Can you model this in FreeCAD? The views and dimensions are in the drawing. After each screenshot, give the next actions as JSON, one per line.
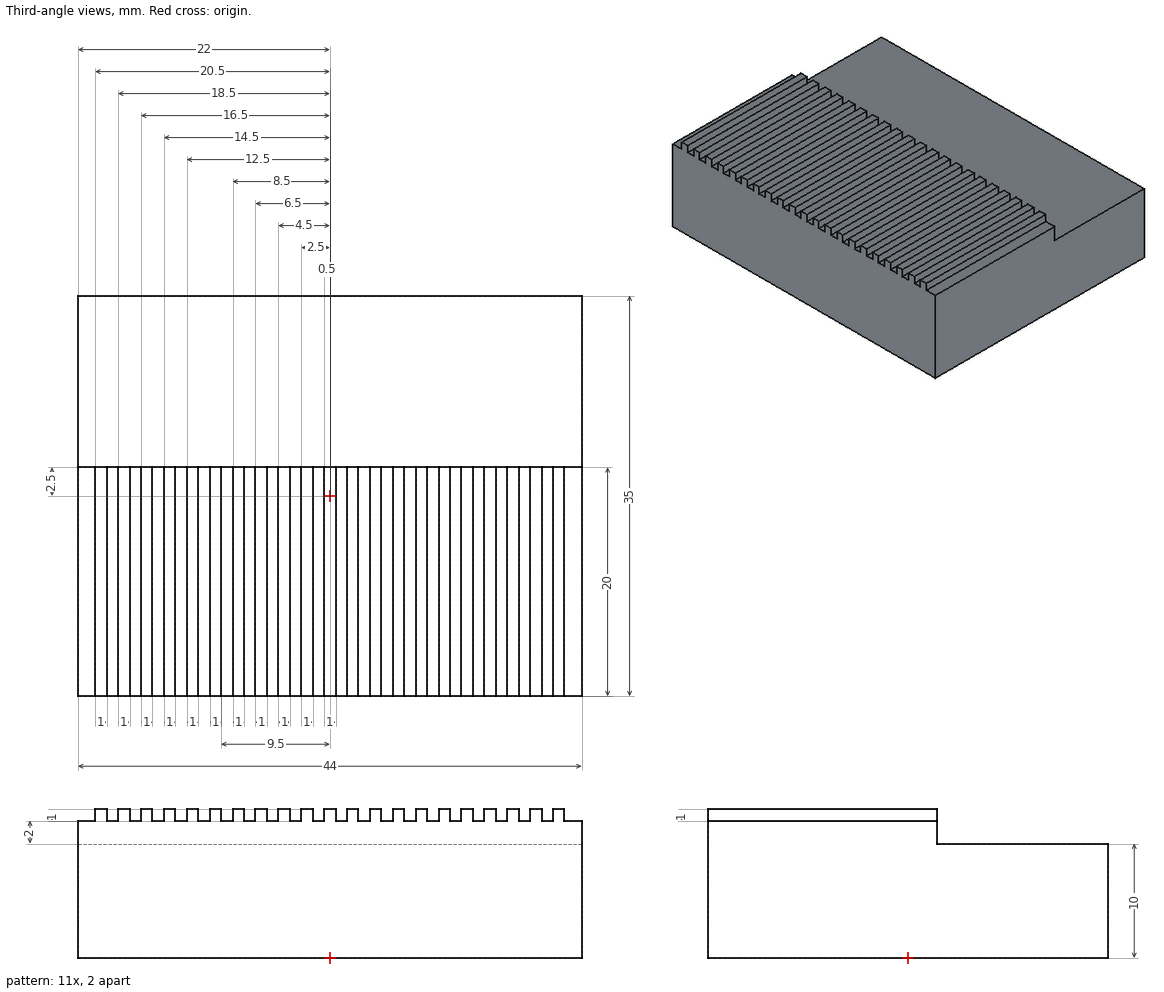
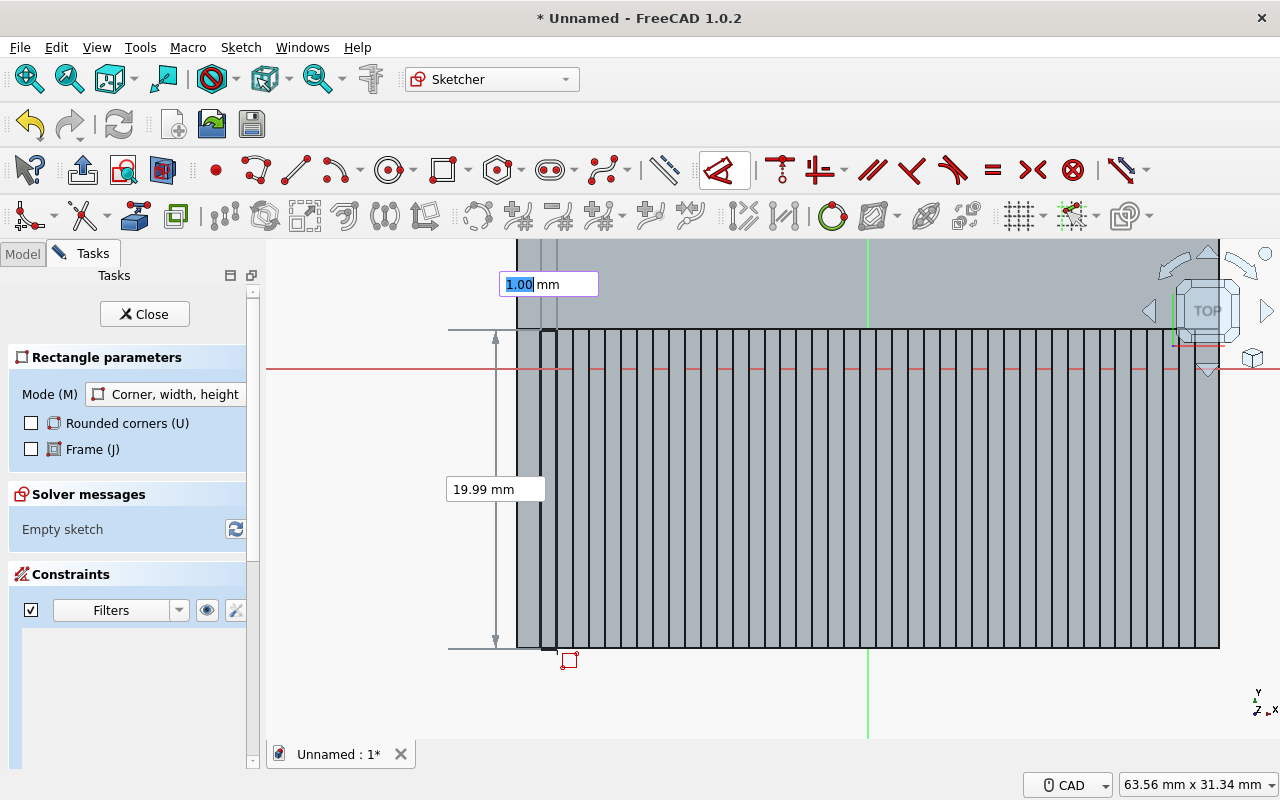
{"action": "type", "text": "1"}
{"action": "key", "text": "Tab"}
{"action": "type", "text": "20"}
{"action": "key", "text": "Return"}
{"action": "key", "text": "Escape"}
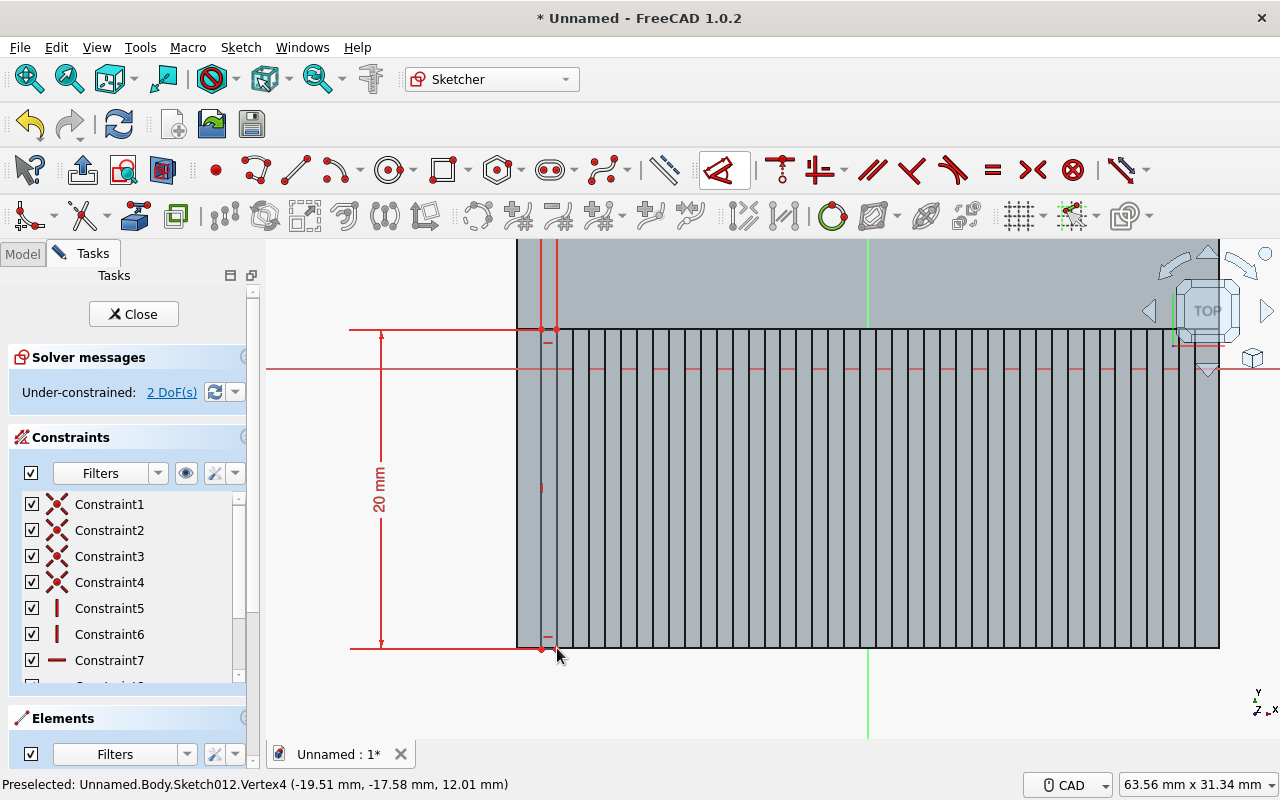
{"action": "left_click", "coordinate": [541, 330]}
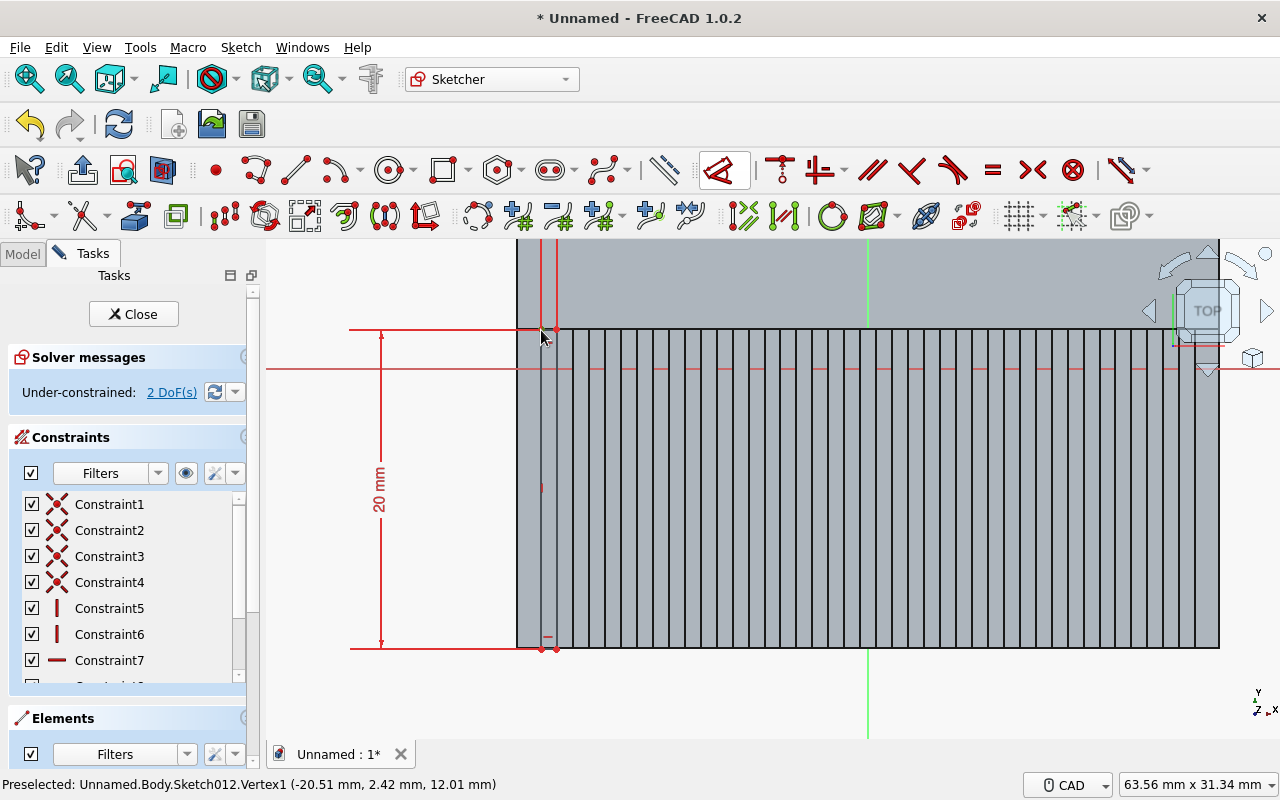
{"action": "key", "text": "i"}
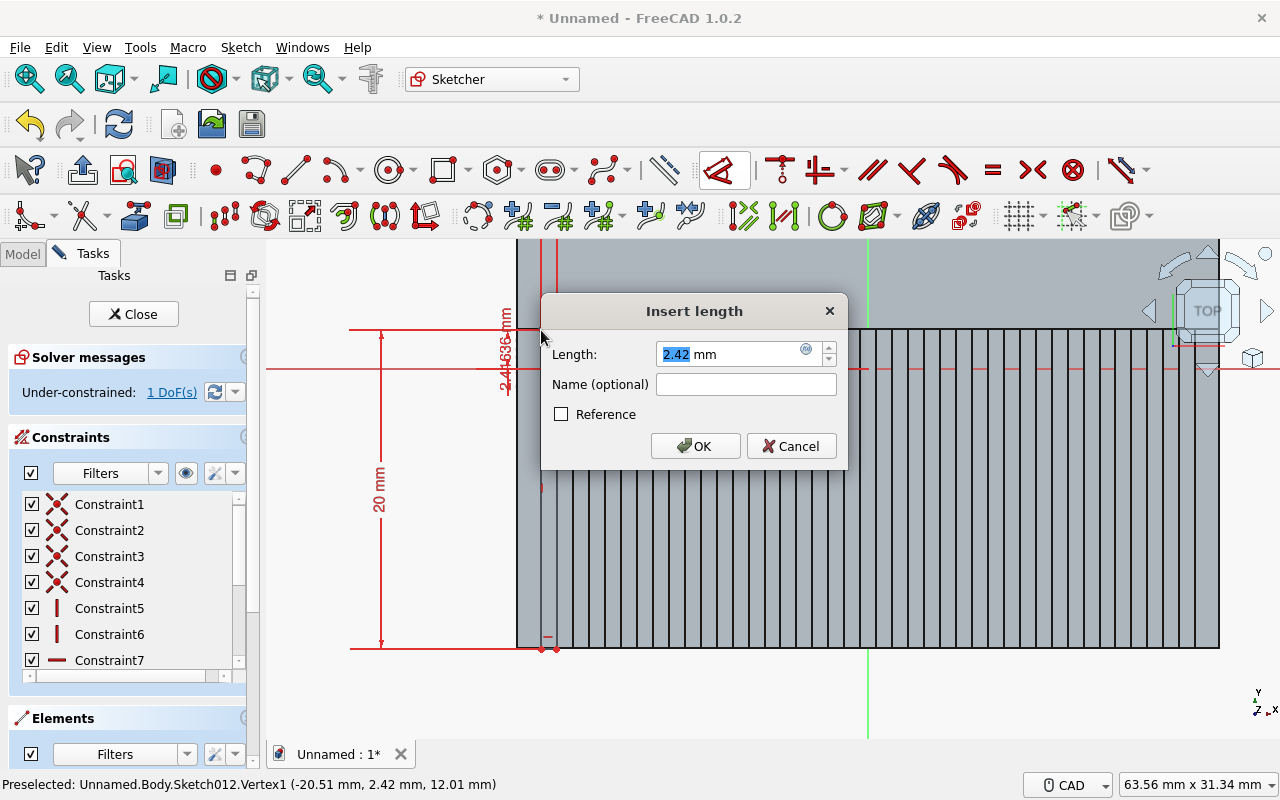
{"action": "type", "text": "2.5"}
{"action": "key", "text": "Return"}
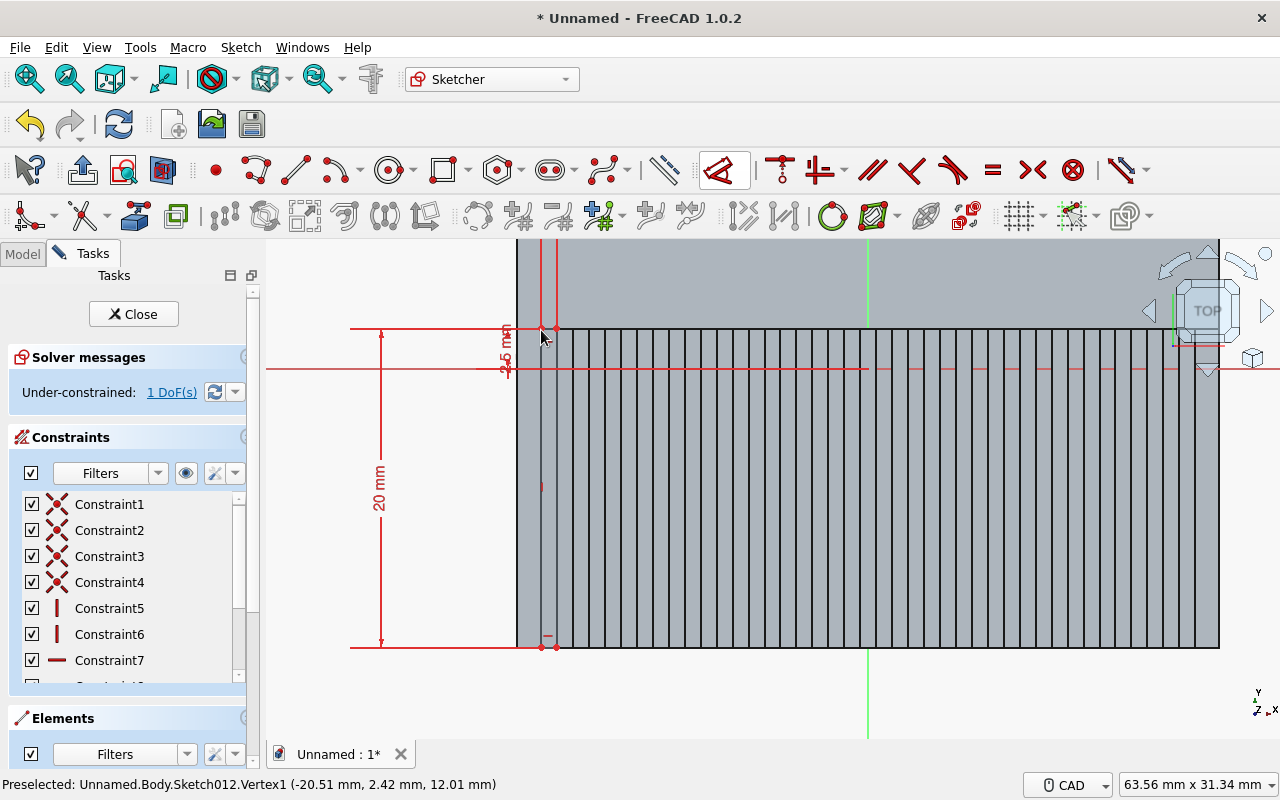
{"action": "left_click", "coordinate": [541, 329]}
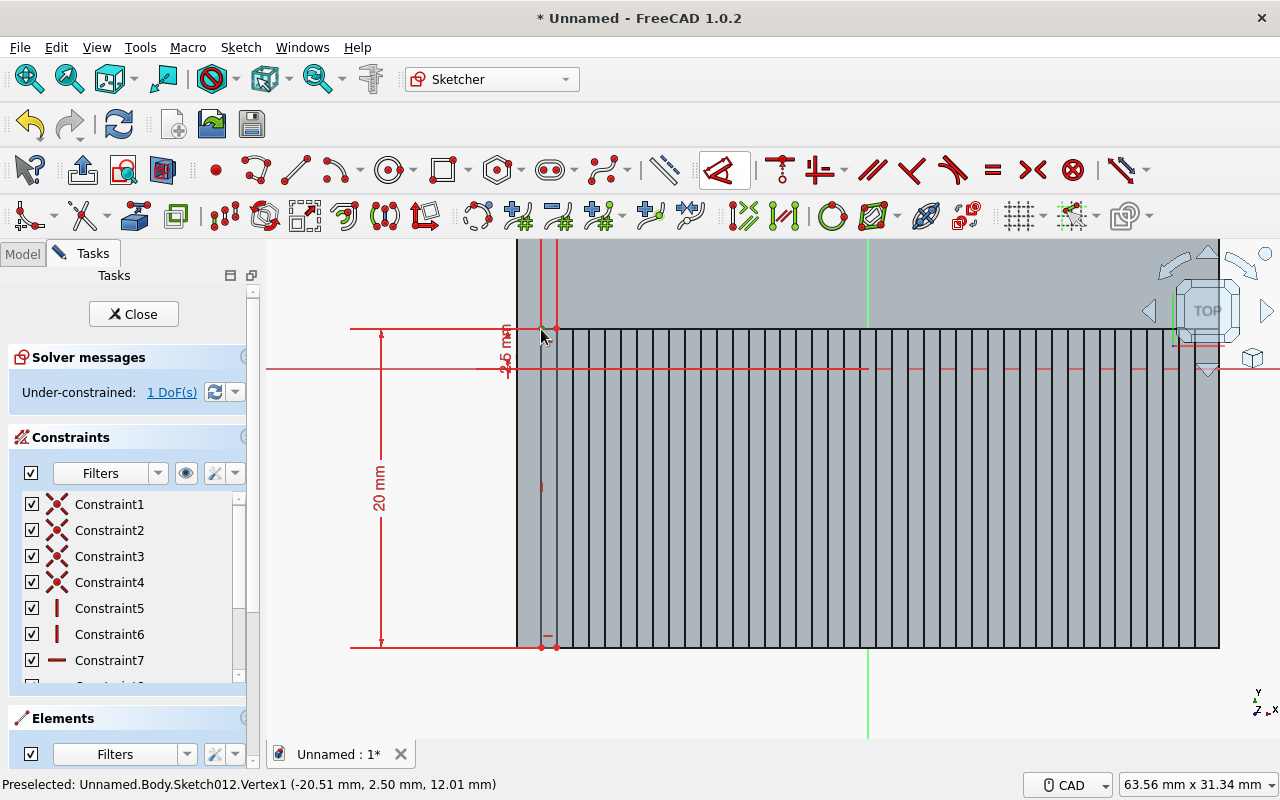
{"action": "key", "text": "l"}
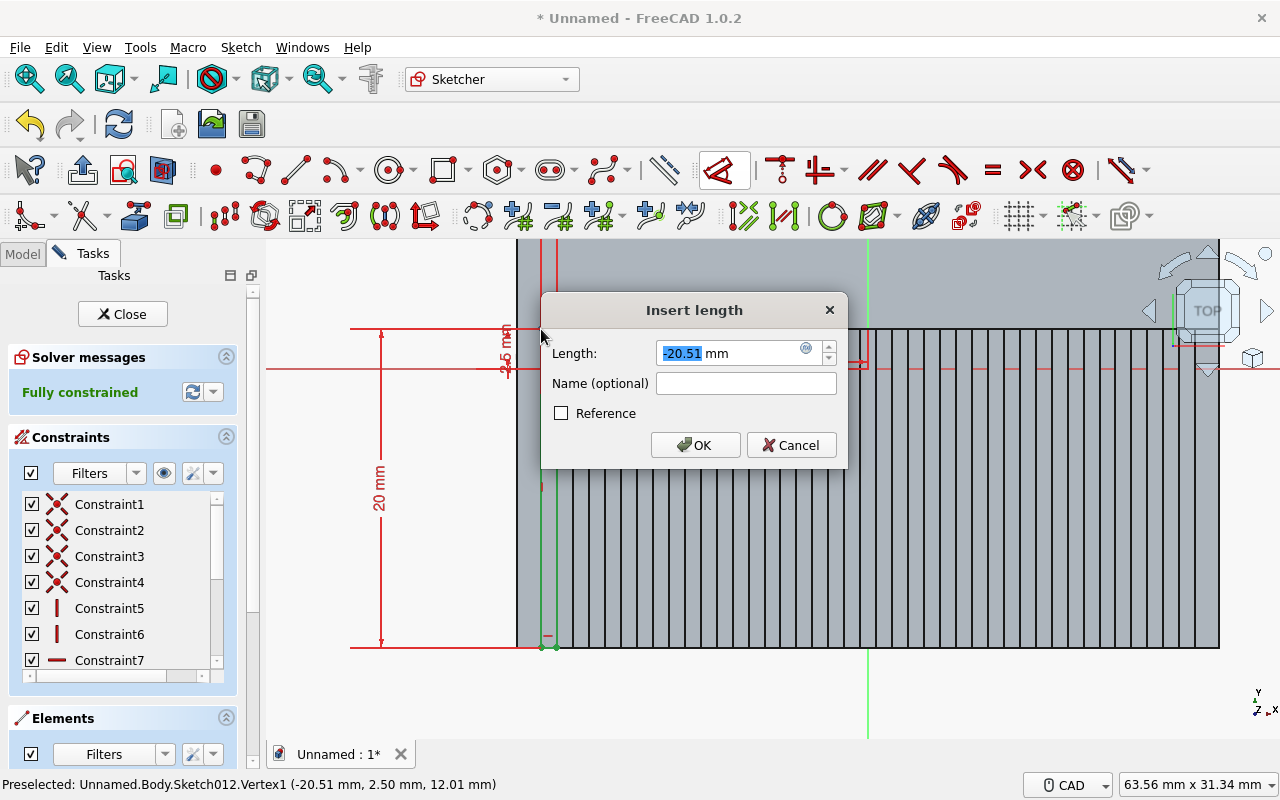
{"action": "type", "text": "-20.5"}
{"action": "key", "text": "Return"}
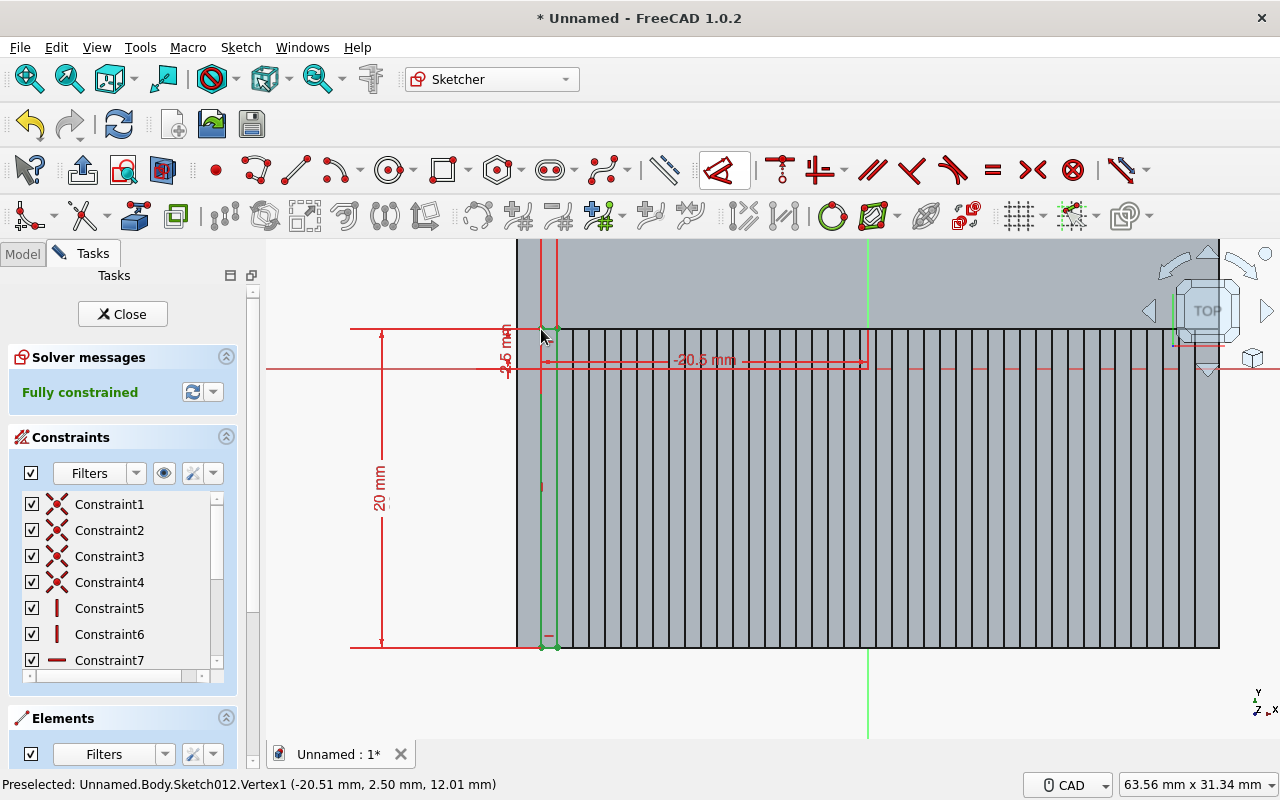
{"action": "left_click", "coordinate": [123, 314]}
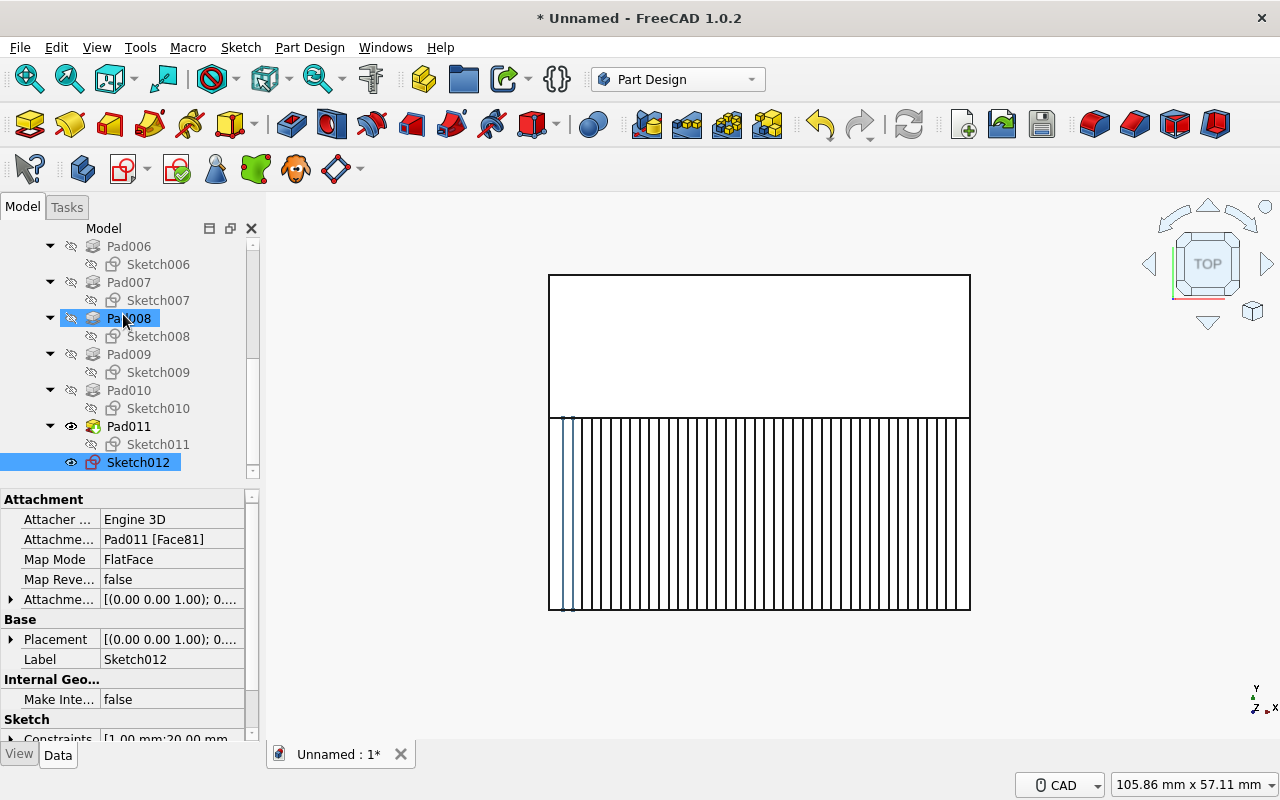
{"action": "left_click", "coordinate": [30, 124]}